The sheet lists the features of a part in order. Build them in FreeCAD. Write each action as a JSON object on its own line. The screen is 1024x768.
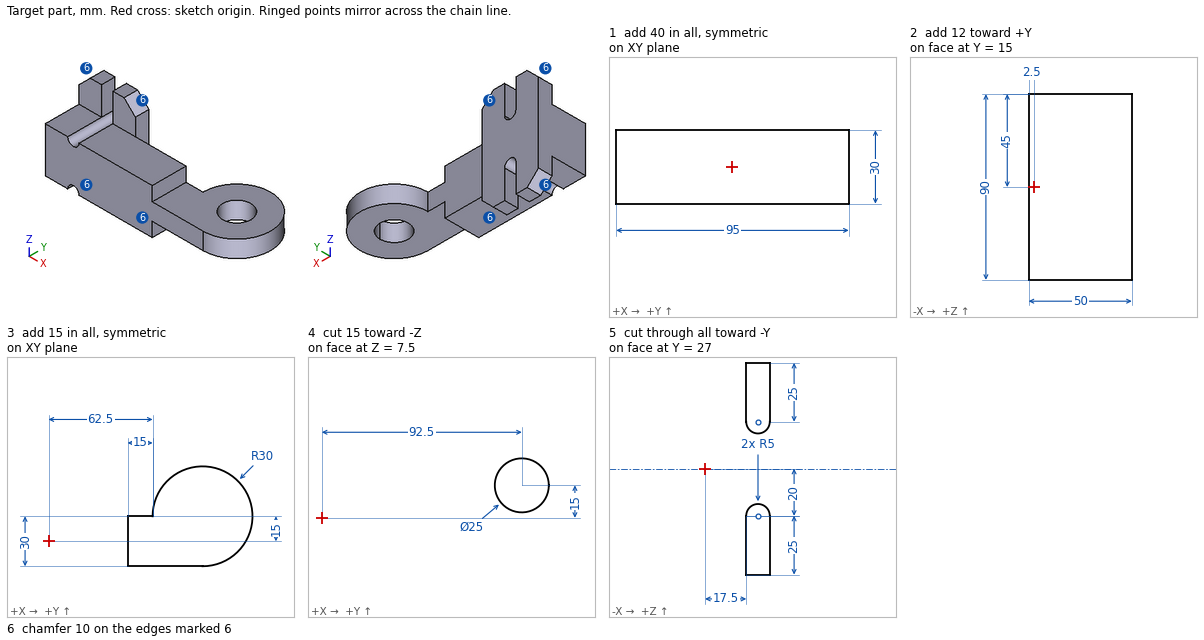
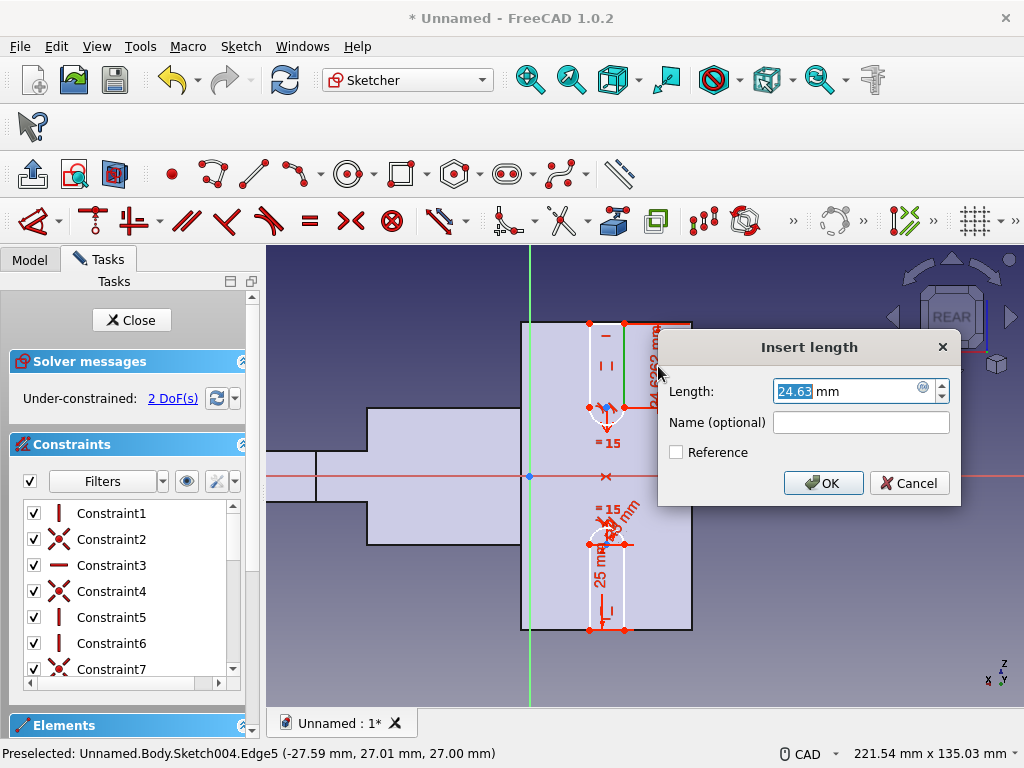
{"action": "type", "text": "25"}
{"action": "key", "text": "Return"}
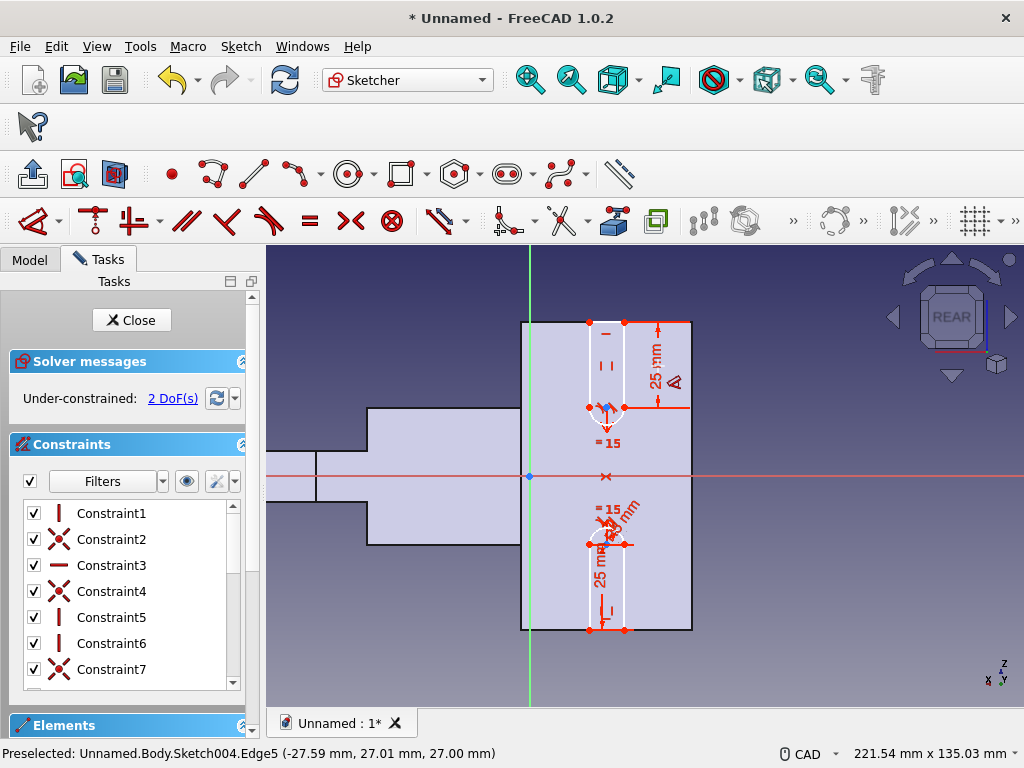
{"action": "left_click", "coordinate": [590, 545]}
{"action": "left_click", "coordinate": [496, 511]}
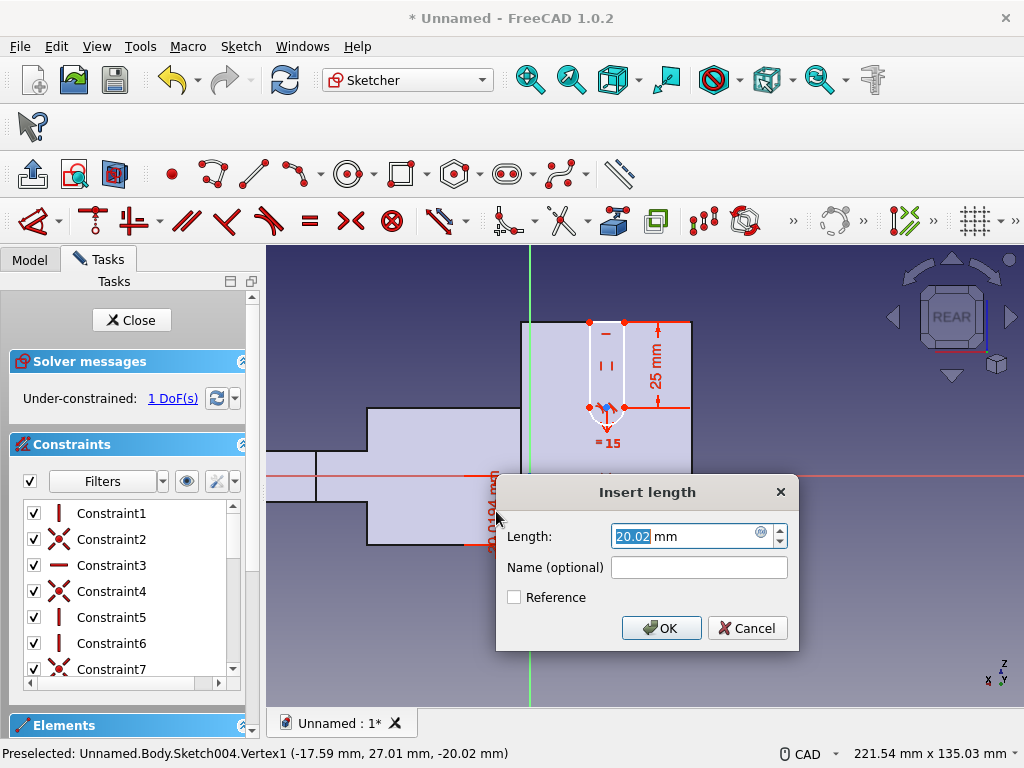
{"action": "type", "text": "20"}
{"action": "key", "text": "Return"}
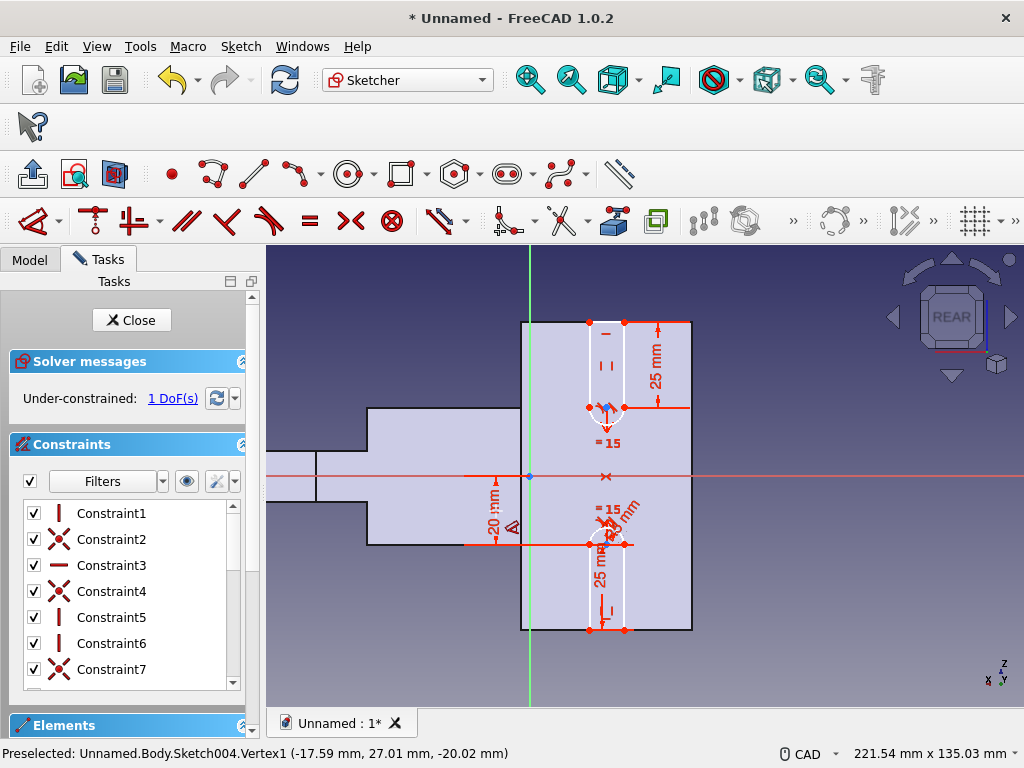
{"action": "left_click", "coordinate": [590, 545]}
{"action": "left_click", "coordinate": [560, 442]}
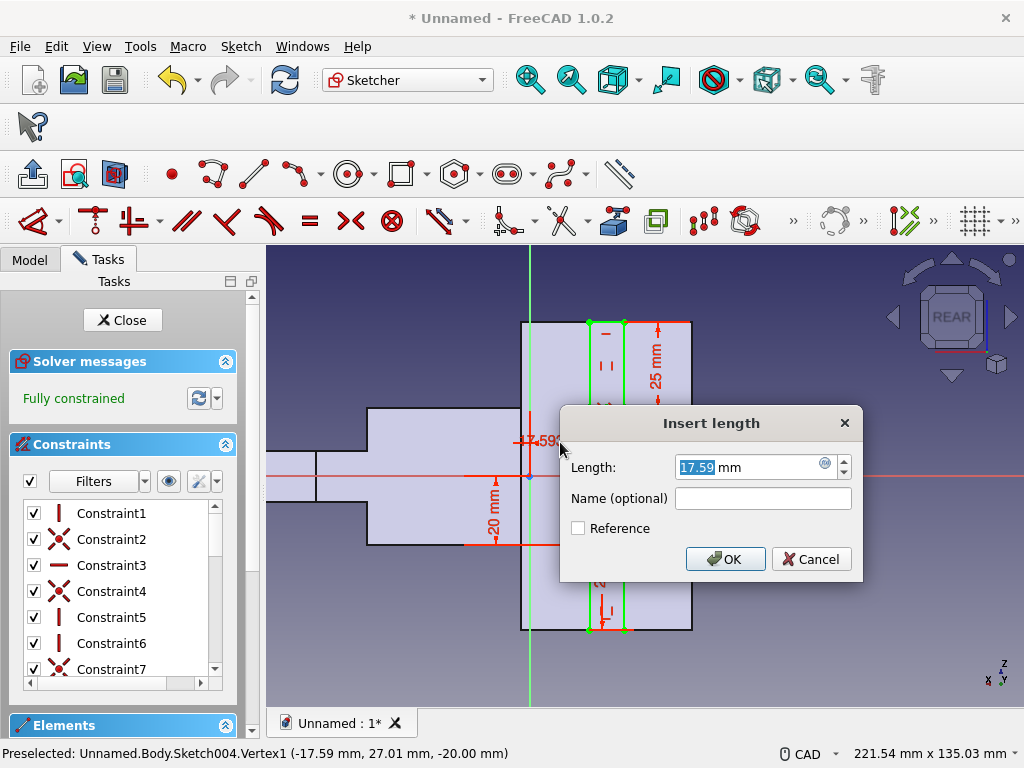
{"action": "type", "text": "17.5"}
{"action": "key", "text": "Return"}
{"action": "key", "text": "Escape"}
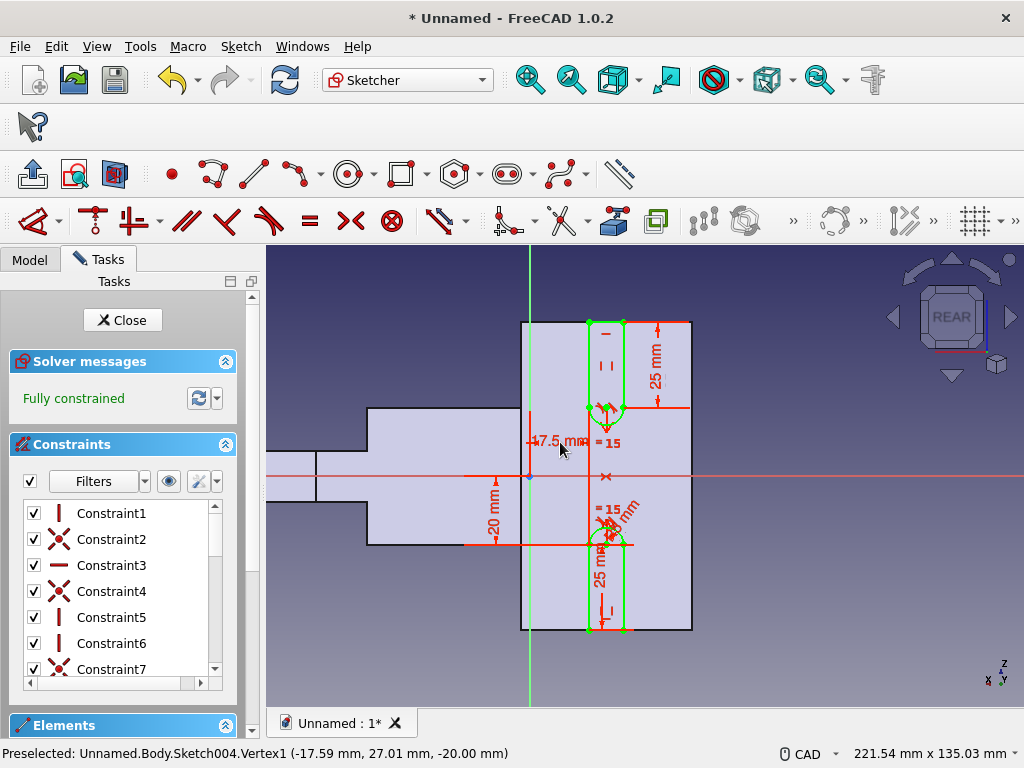
{"action": "left_click", "coordinate": [123, 320]}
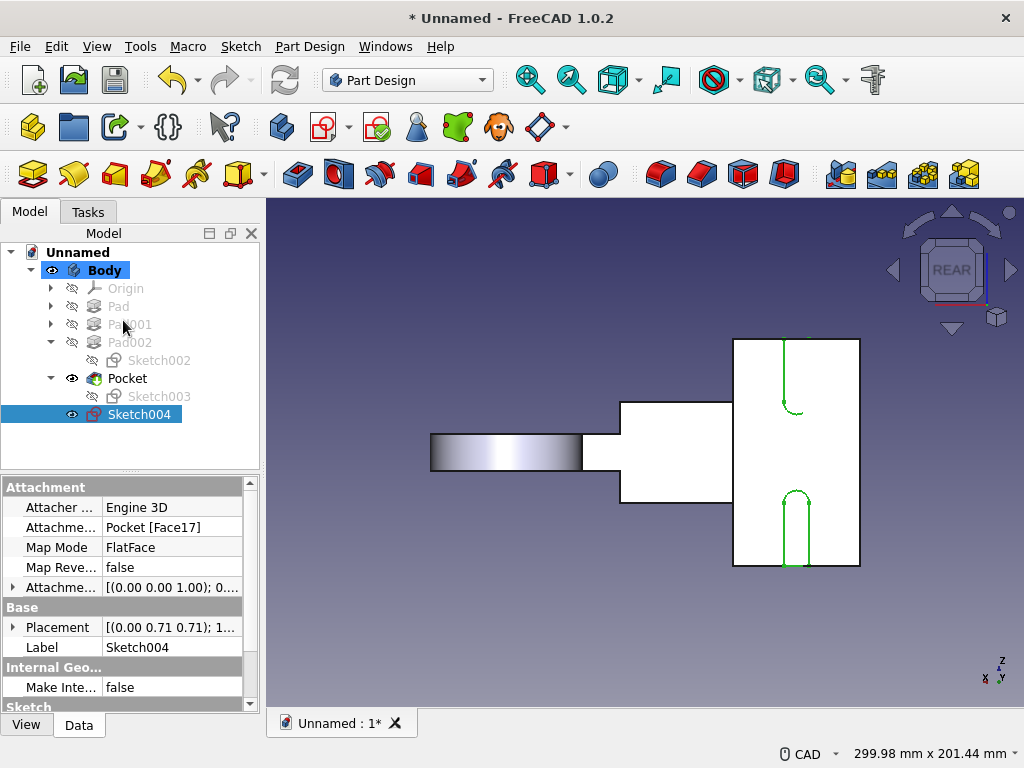
{"action": "left_click", "coordinate": [298, 174]}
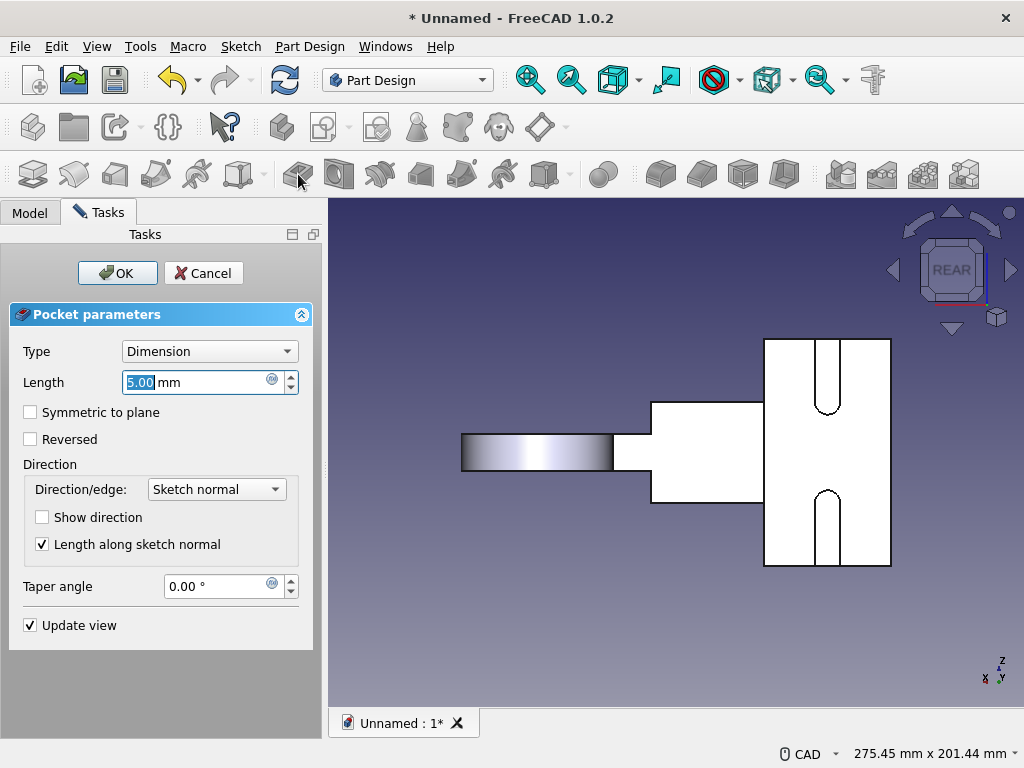
{"action": "left_click", "coordinate": [210, 352]}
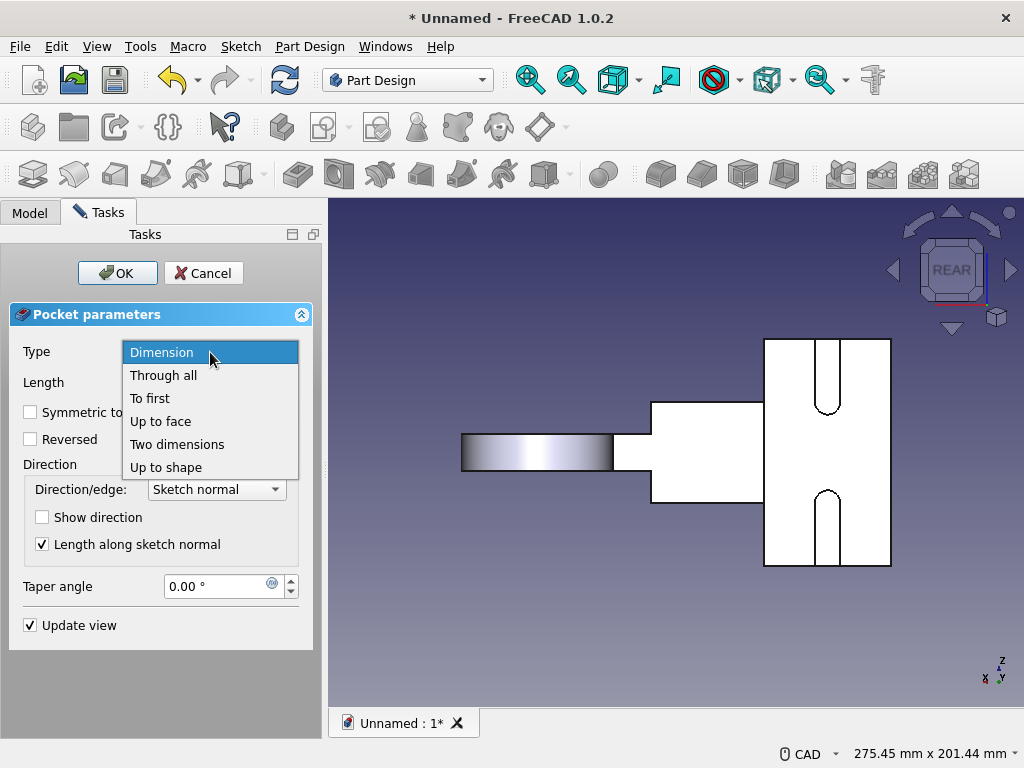
{"action": "left_click", "coordinate": [208, 376]}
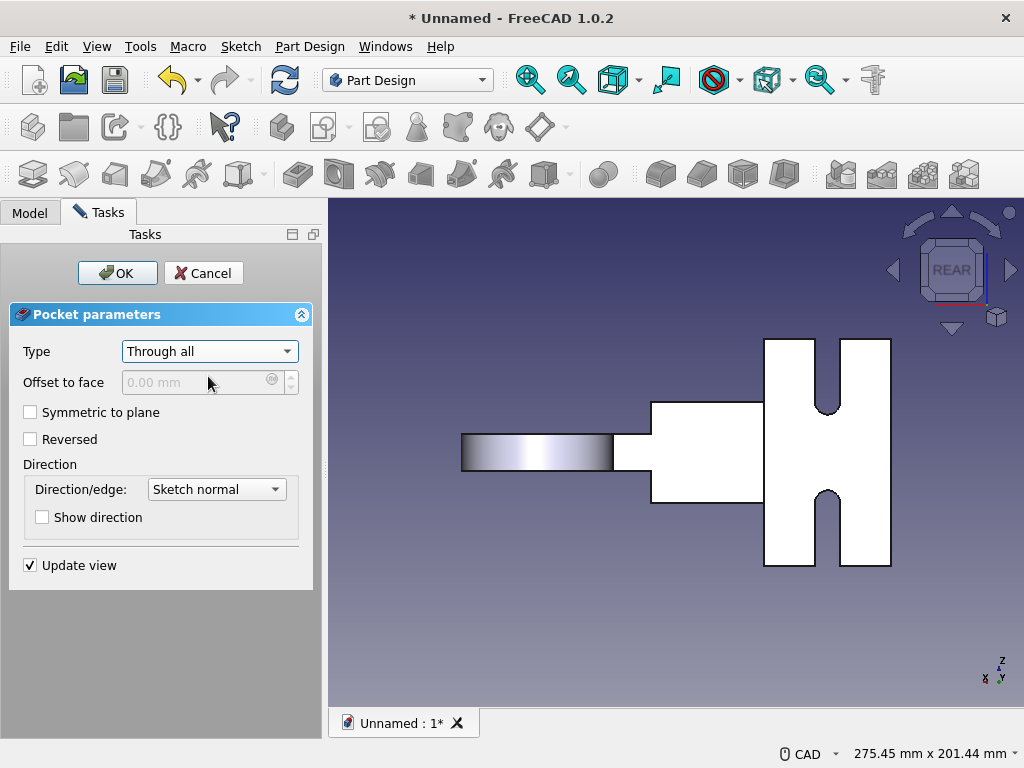
{"action": "left_click", "coordinate": [118, 273]}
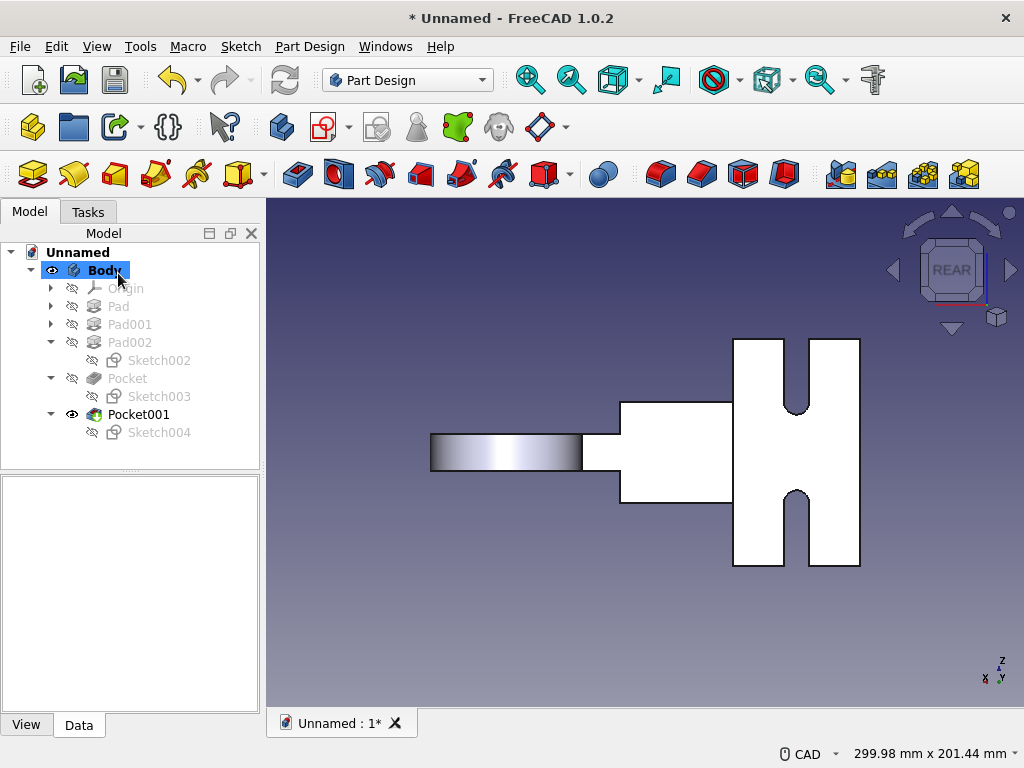
{"action": "key", "text": "0"}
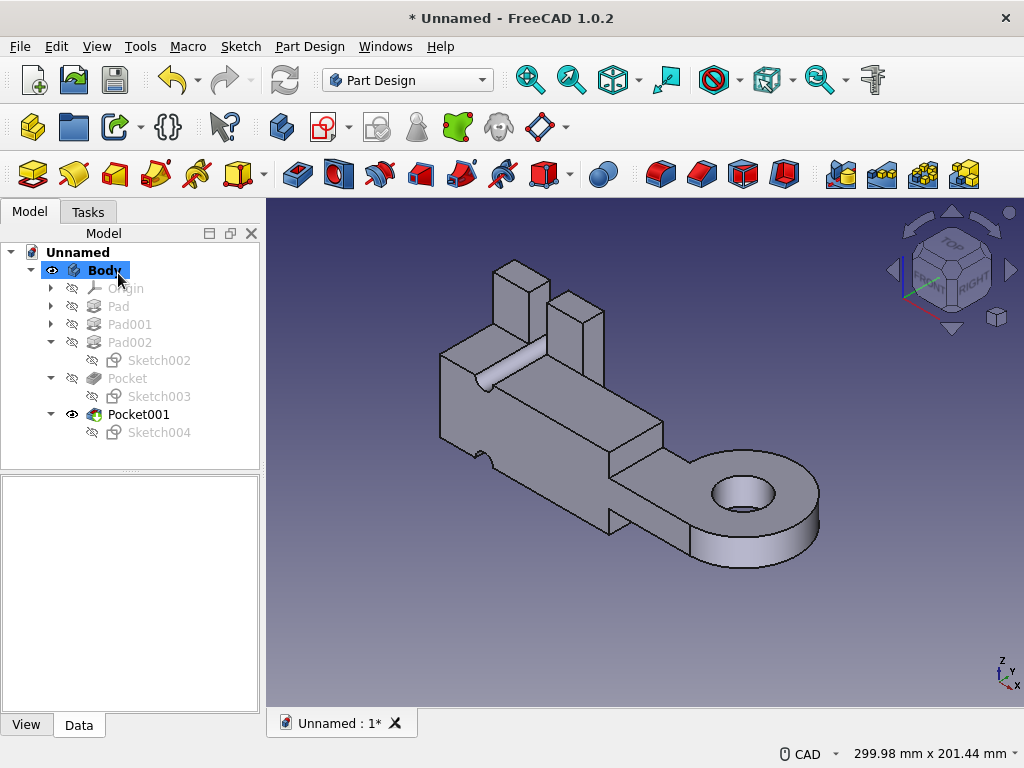
{"action": "left_click", "coordinate": [593, 316]}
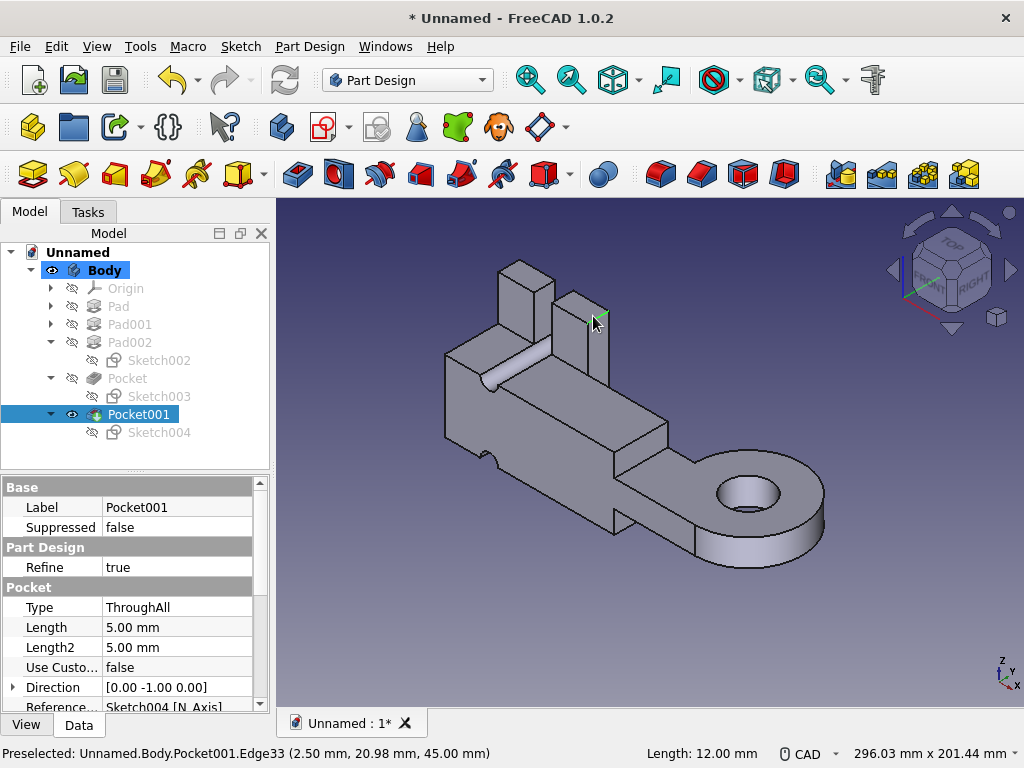
{"action": "key", "text": "2"}